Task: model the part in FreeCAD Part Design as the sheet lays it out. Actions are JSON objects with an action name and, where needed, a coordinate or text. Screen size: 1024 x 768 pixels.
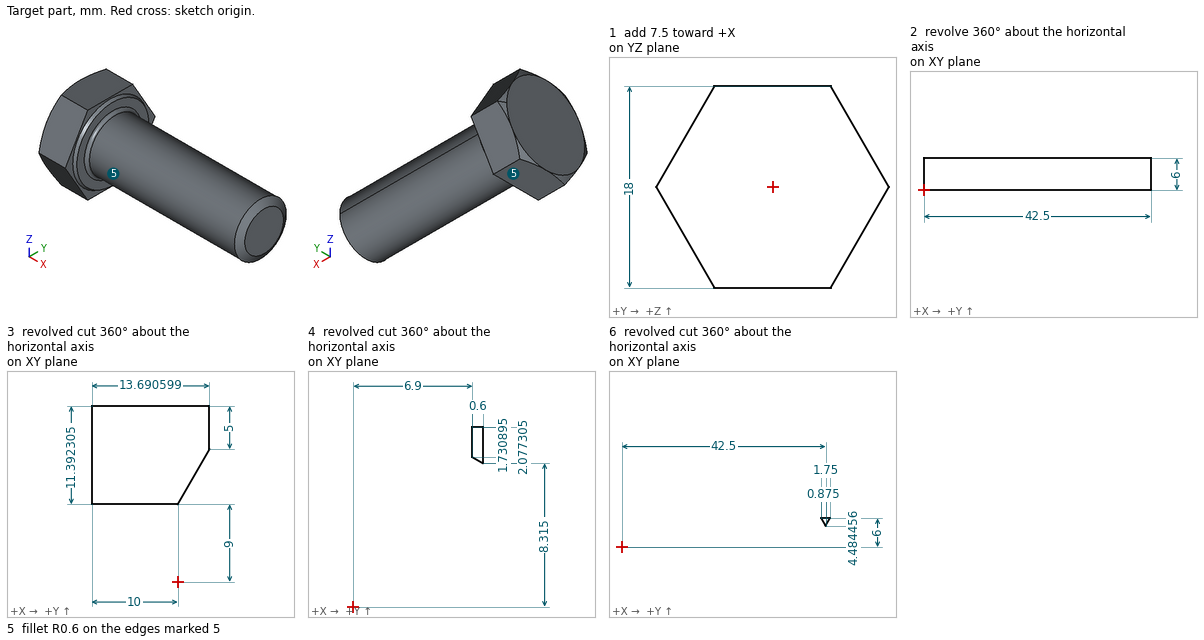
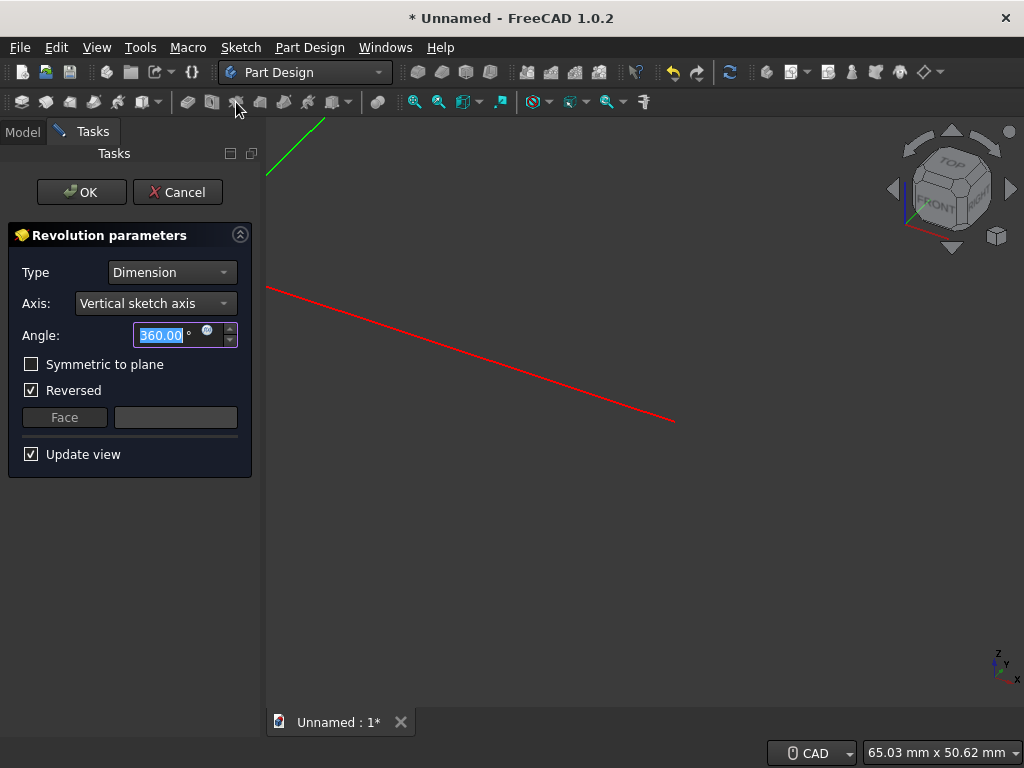
{"action": "left_click", "coordinate": [156, 304]}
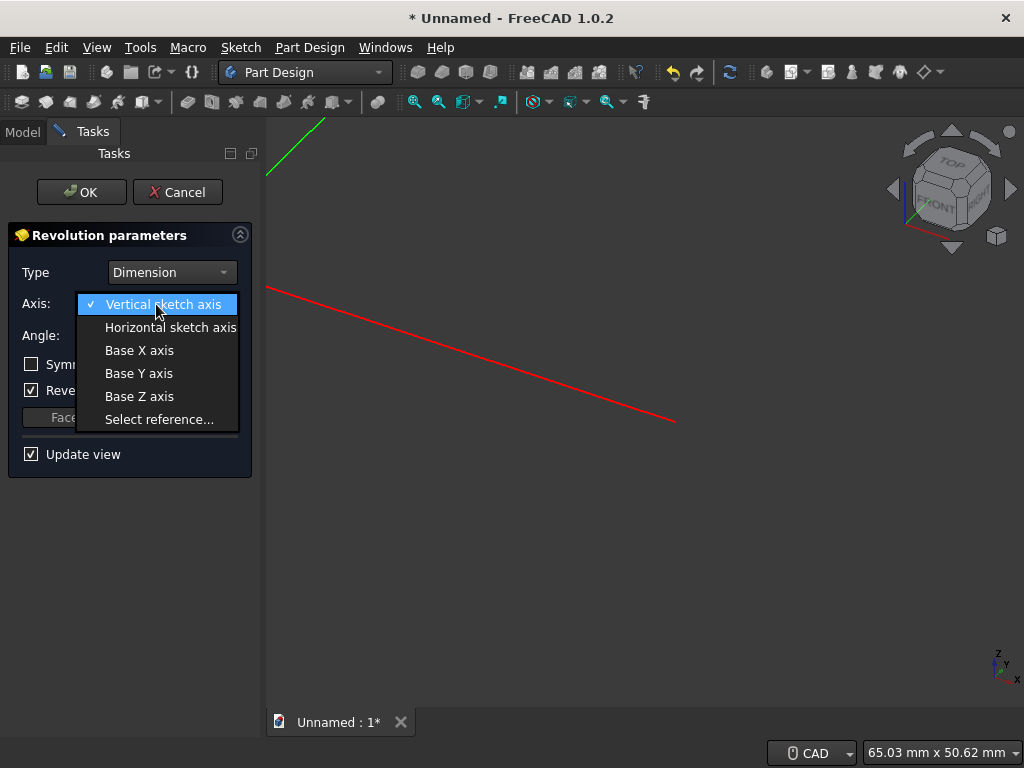
{"action": "left_click", "coordinate": [156, 328]}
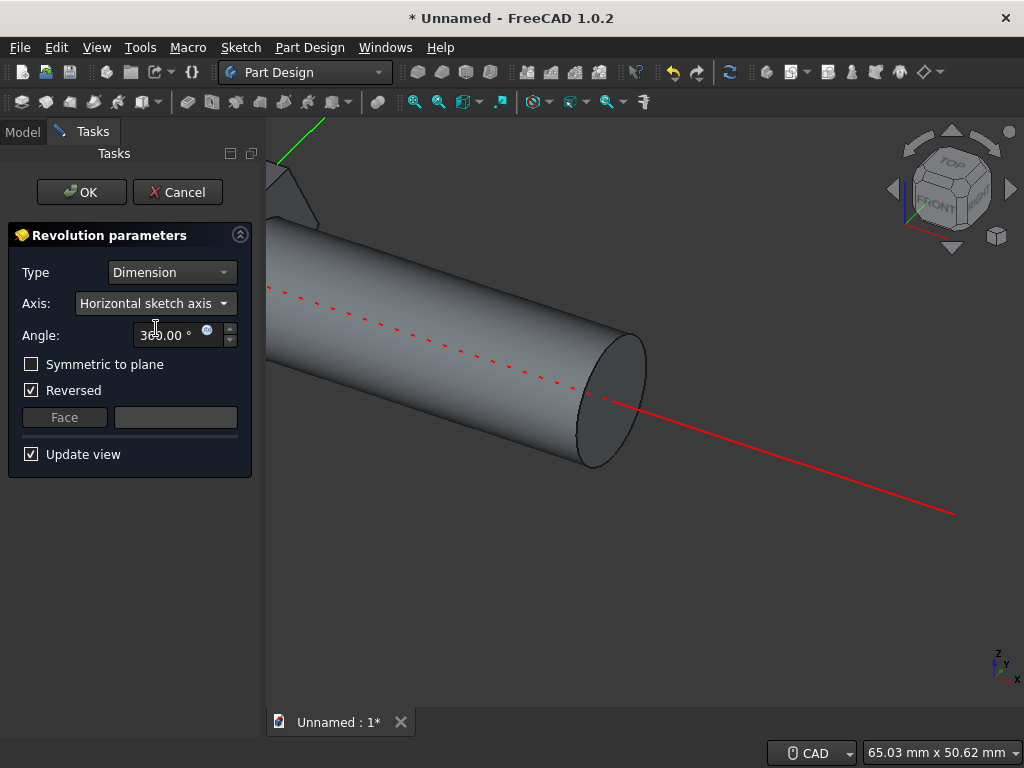
{"action": "left_click", "coordinate": [82, 192]}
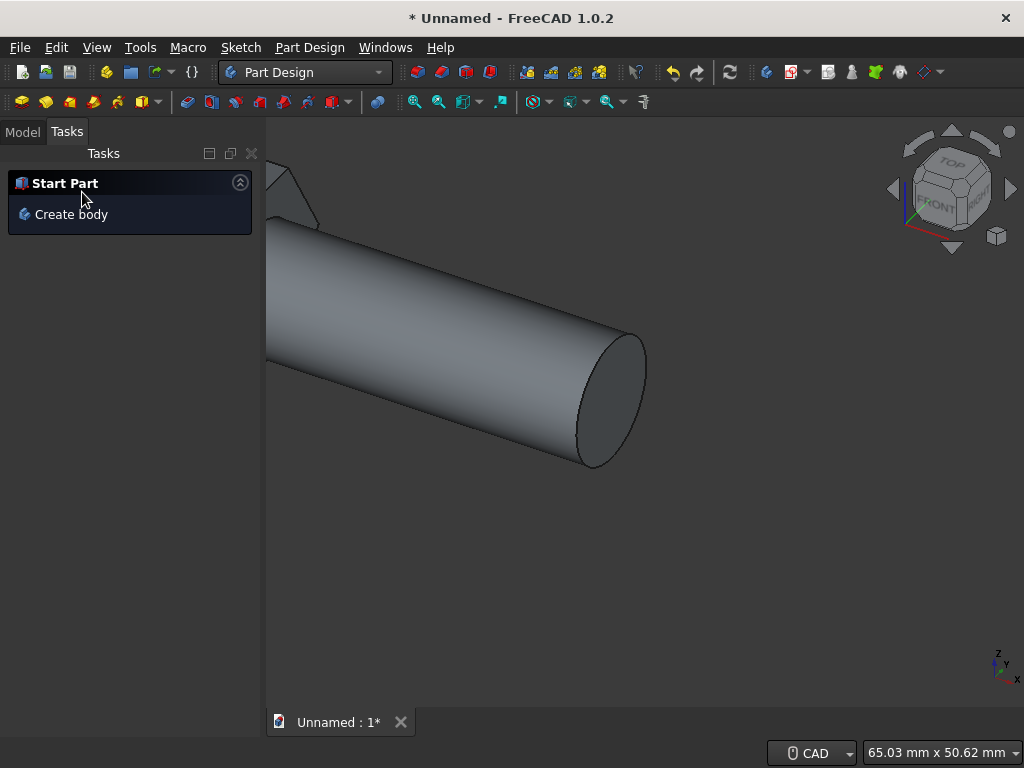
{"action": "left_click", "coordinate": [416, 102]}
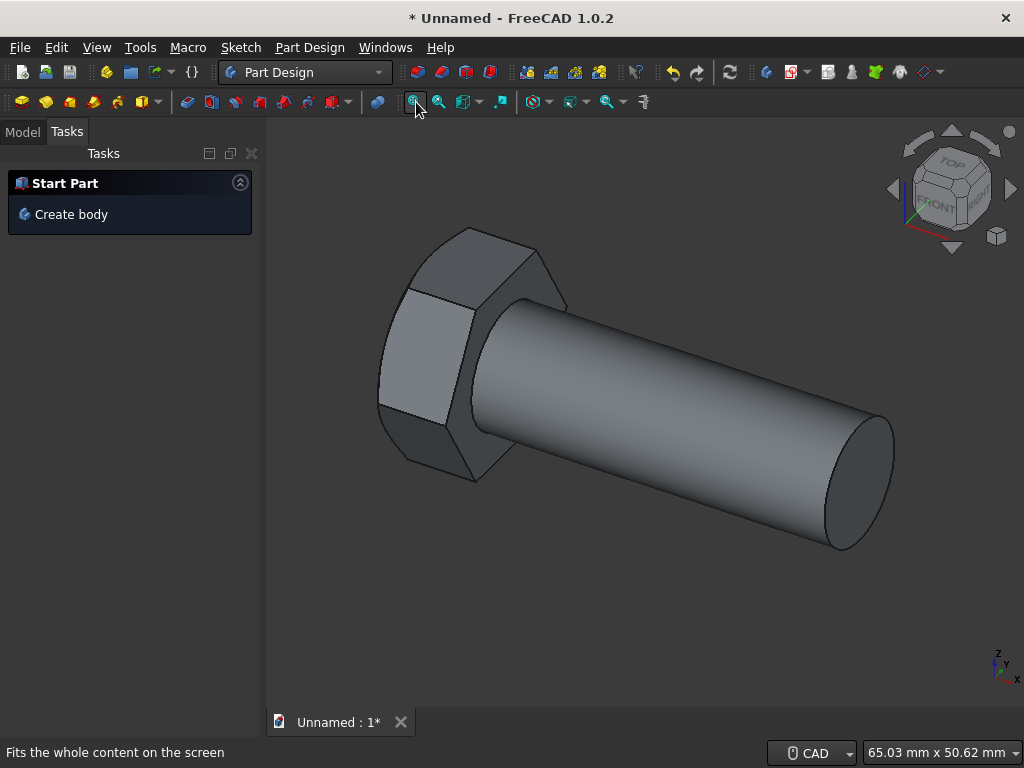
{"action": "left_click", "coordinate": [792, 72]}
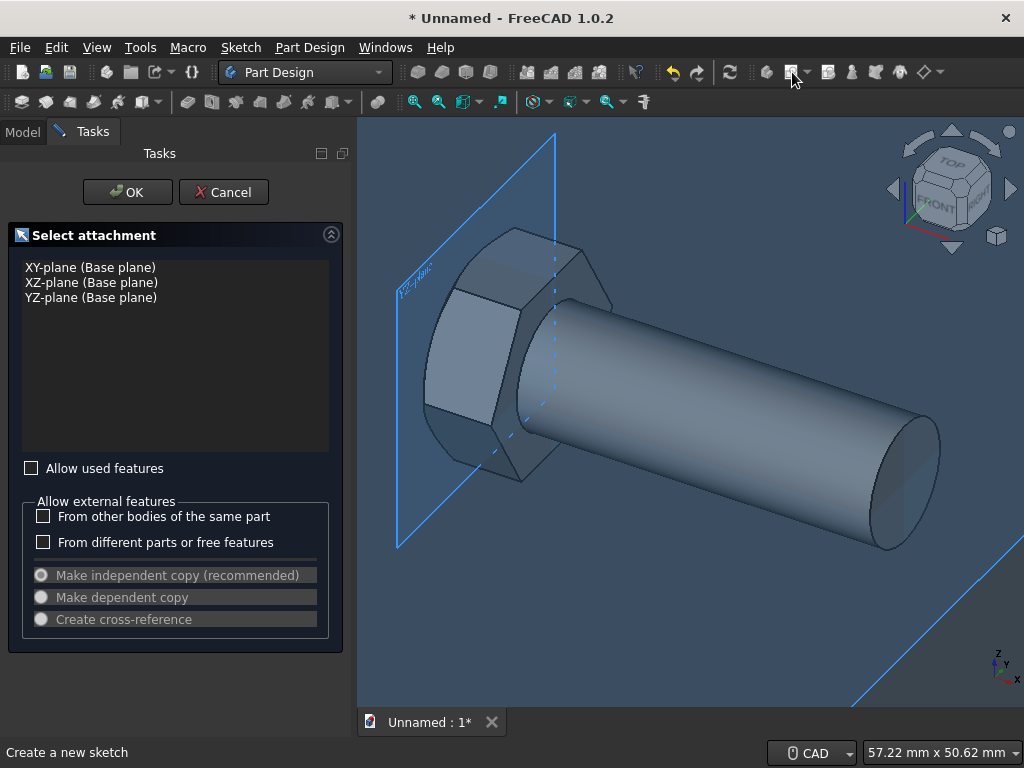
{"action": "left_click", "coordinate": [82, 268]}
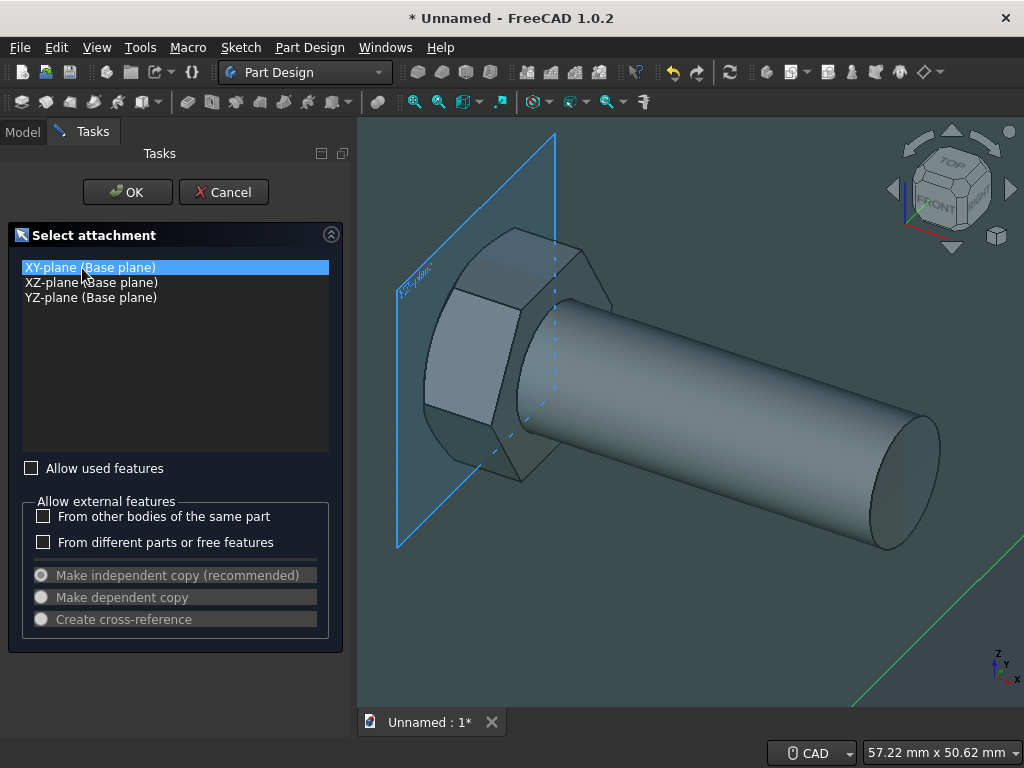
{"action": "left_click", "coordinate": [128, 192]}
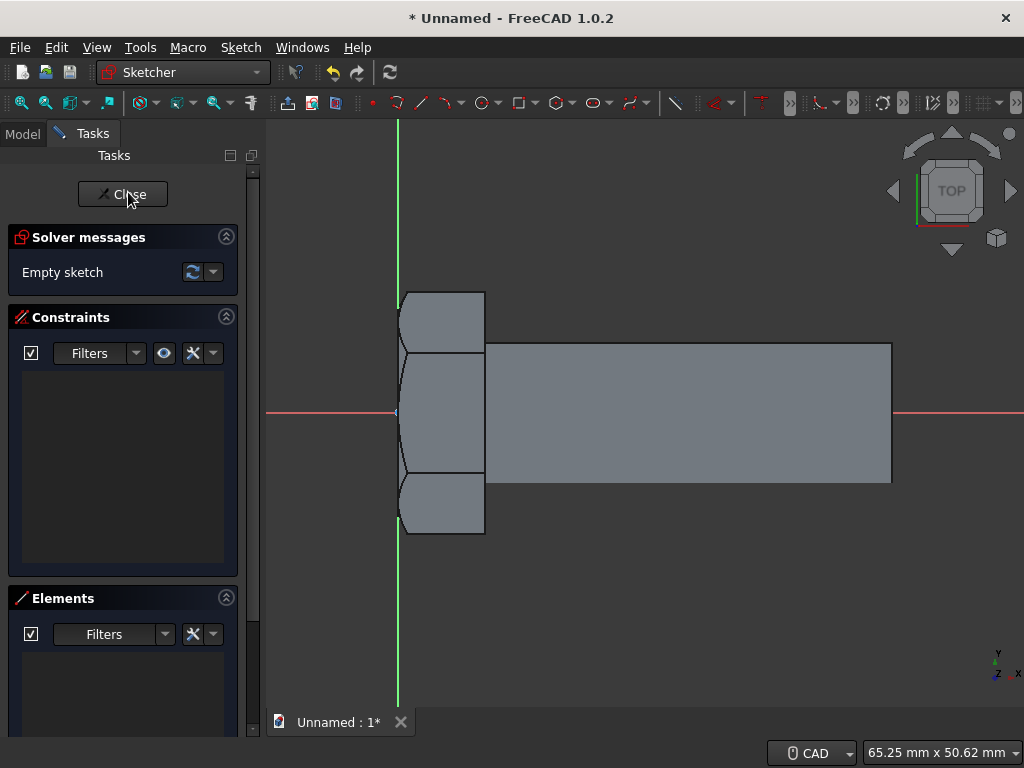
{"action": "left_click", "coordinate": [336, 104]}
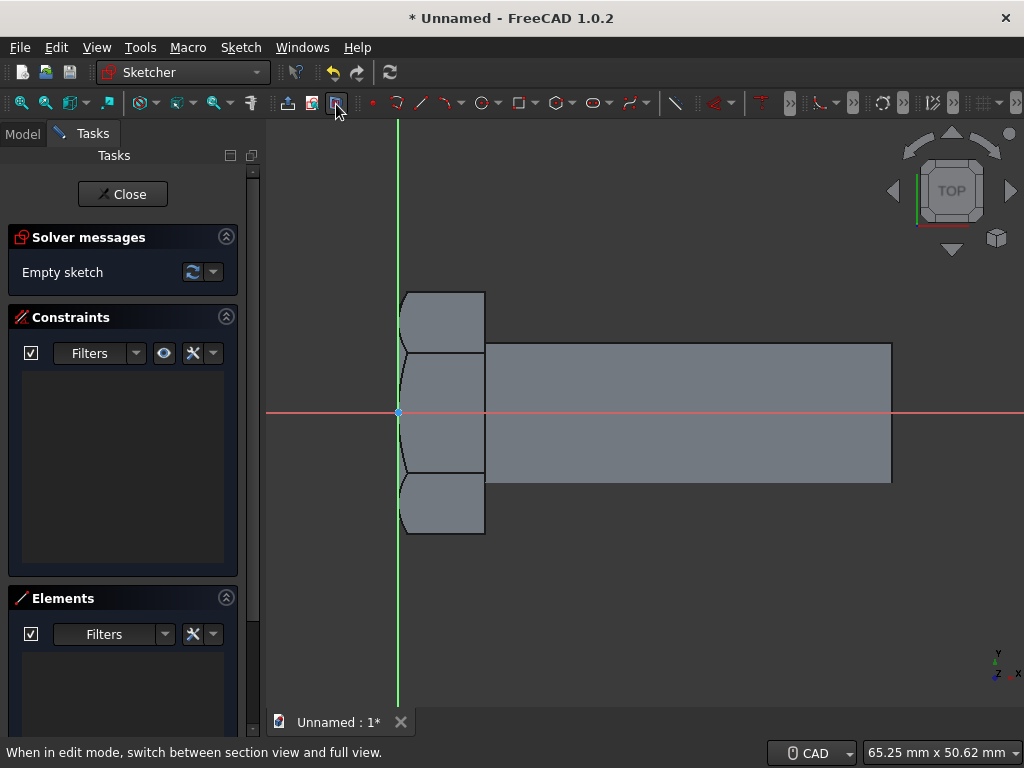
{"action": "scroll", "coordinate": [476, 297], "scroll_direction": "up", "scroll_amount": 14}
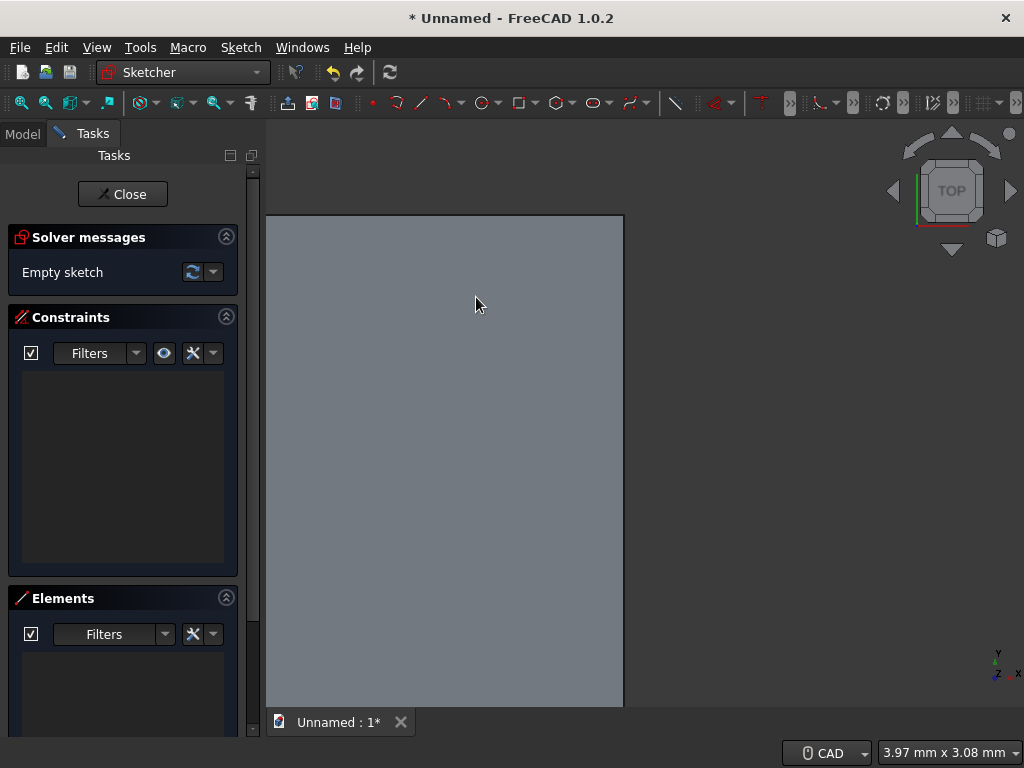
{"action": "left_click", "coordinate": [398, 104]}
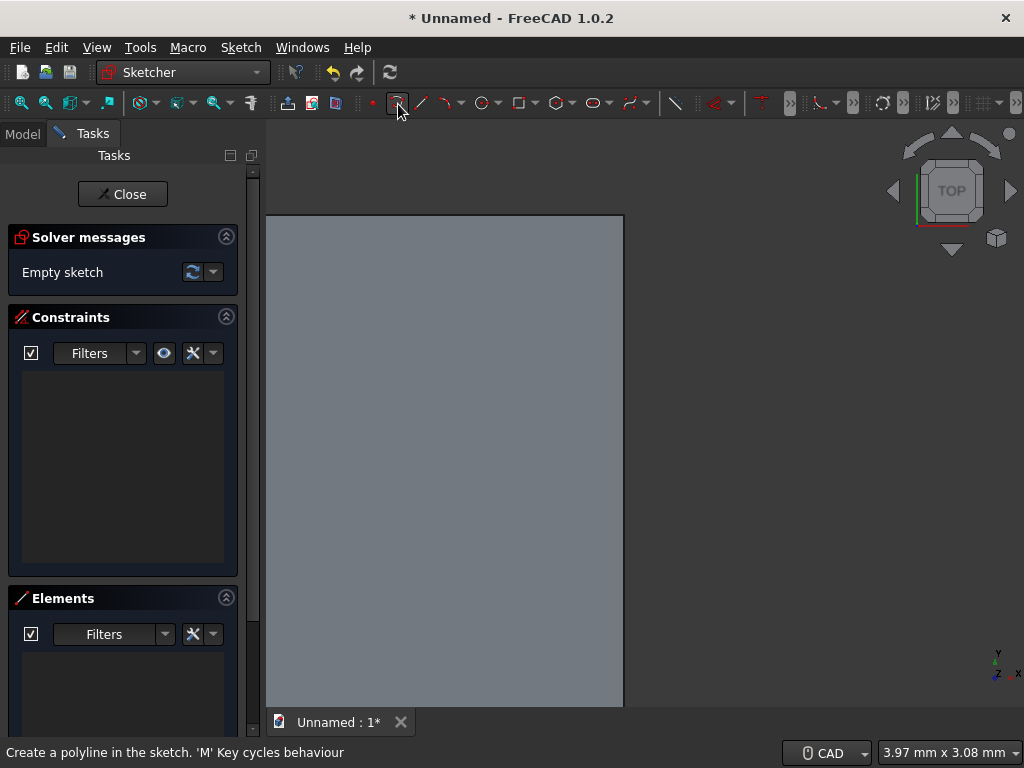
{"action": "left_click", "coordinate": [510, 545]}
{"action": "left_click", "coordinate": [624, 612]}
{"action": "left_click", "coordinate": [624, 215]}
{"action": "left_click", "coordinate": [510, 215]}
{"action": "left_click", "coordinate": [510, 546]}
{"action": "key", "text": "Escape"}
{"action": "key", "text": "Escape"}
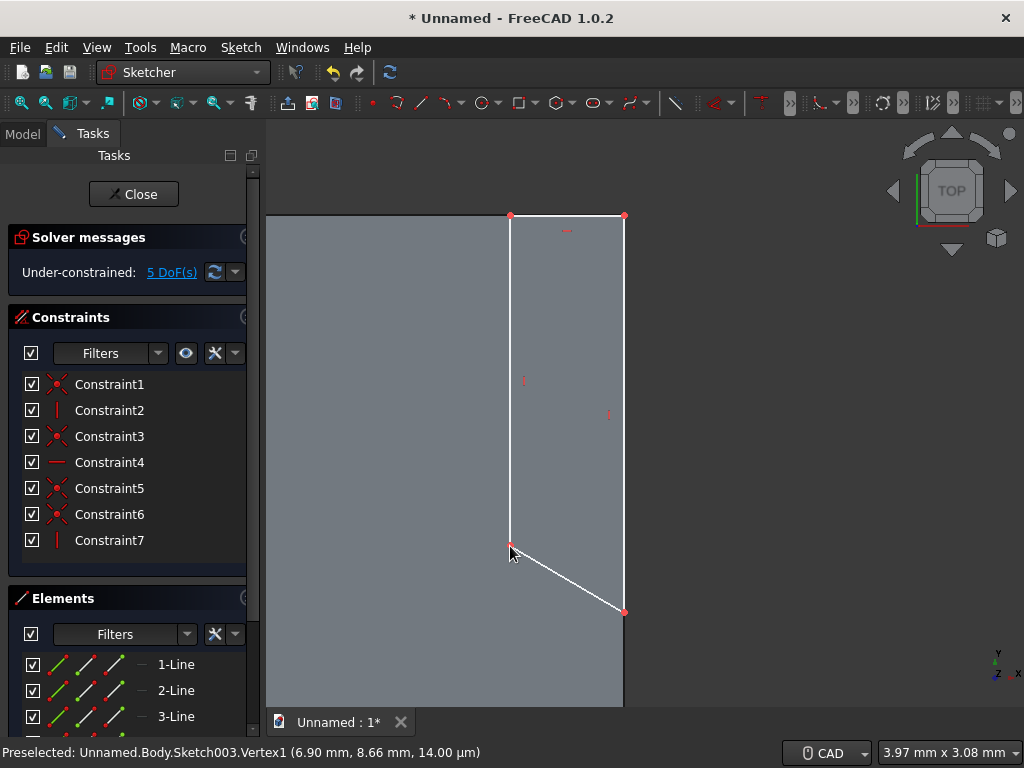
{"action": "left_click", "coordinate": [714, 104]}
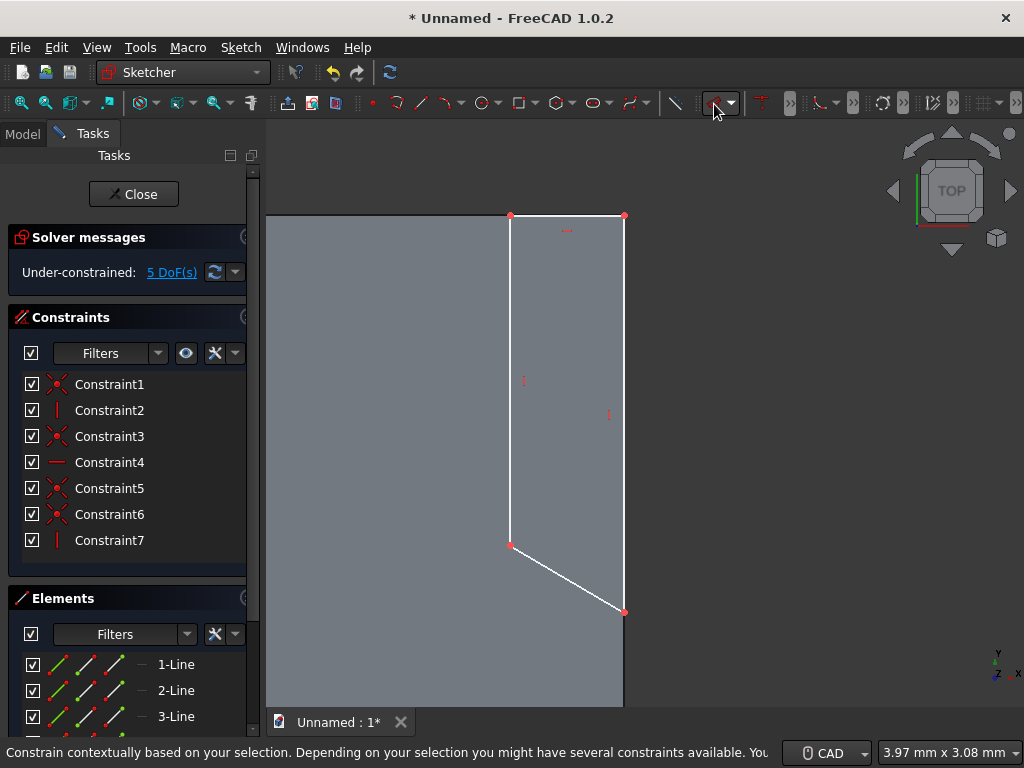
{"action": "left_click", "coordinate": [590, 216]}
{"action": "left_click", "coordinate": [567, 182]}